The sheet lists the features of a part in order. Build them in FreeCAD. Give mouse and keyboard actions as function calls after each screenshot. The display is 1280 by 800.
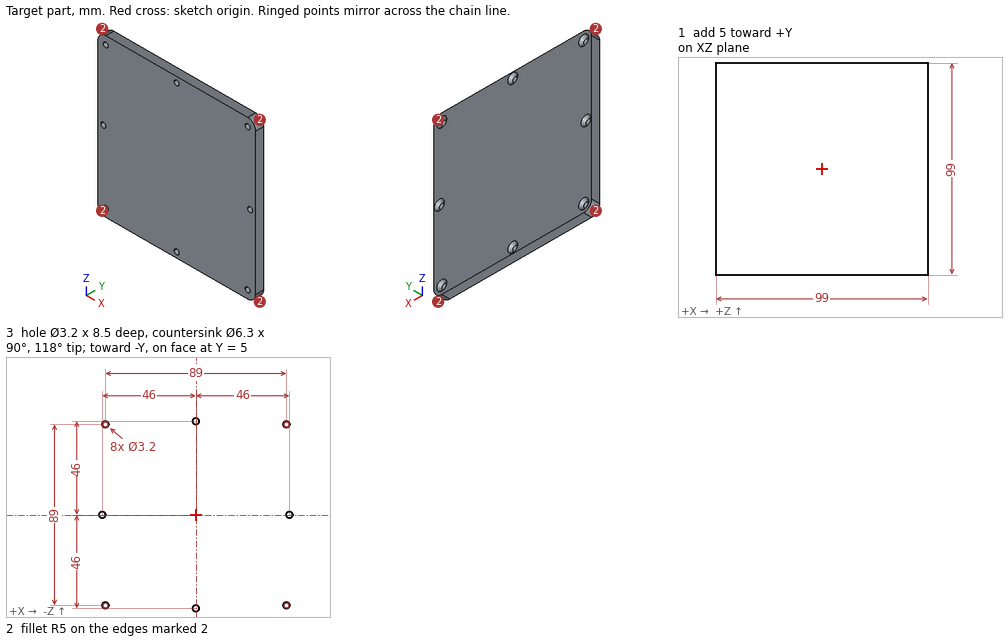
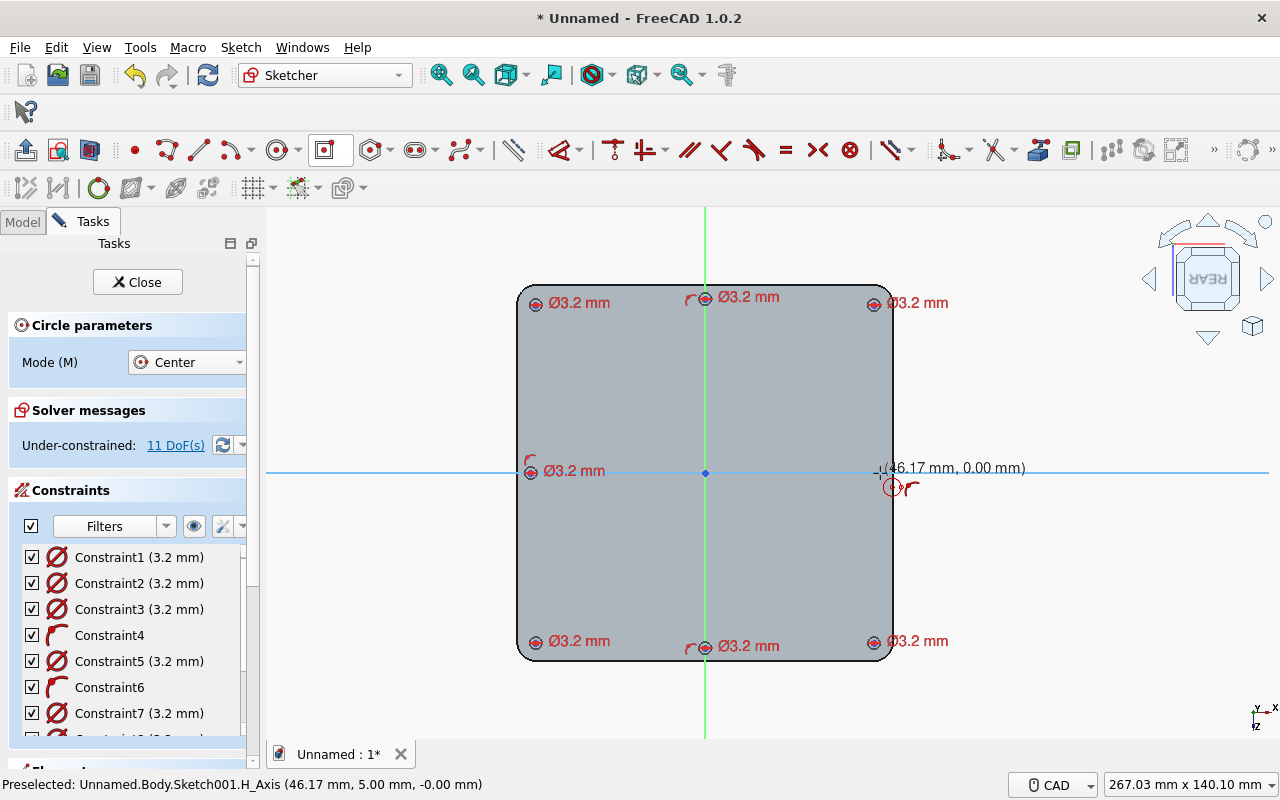
click(880, 473)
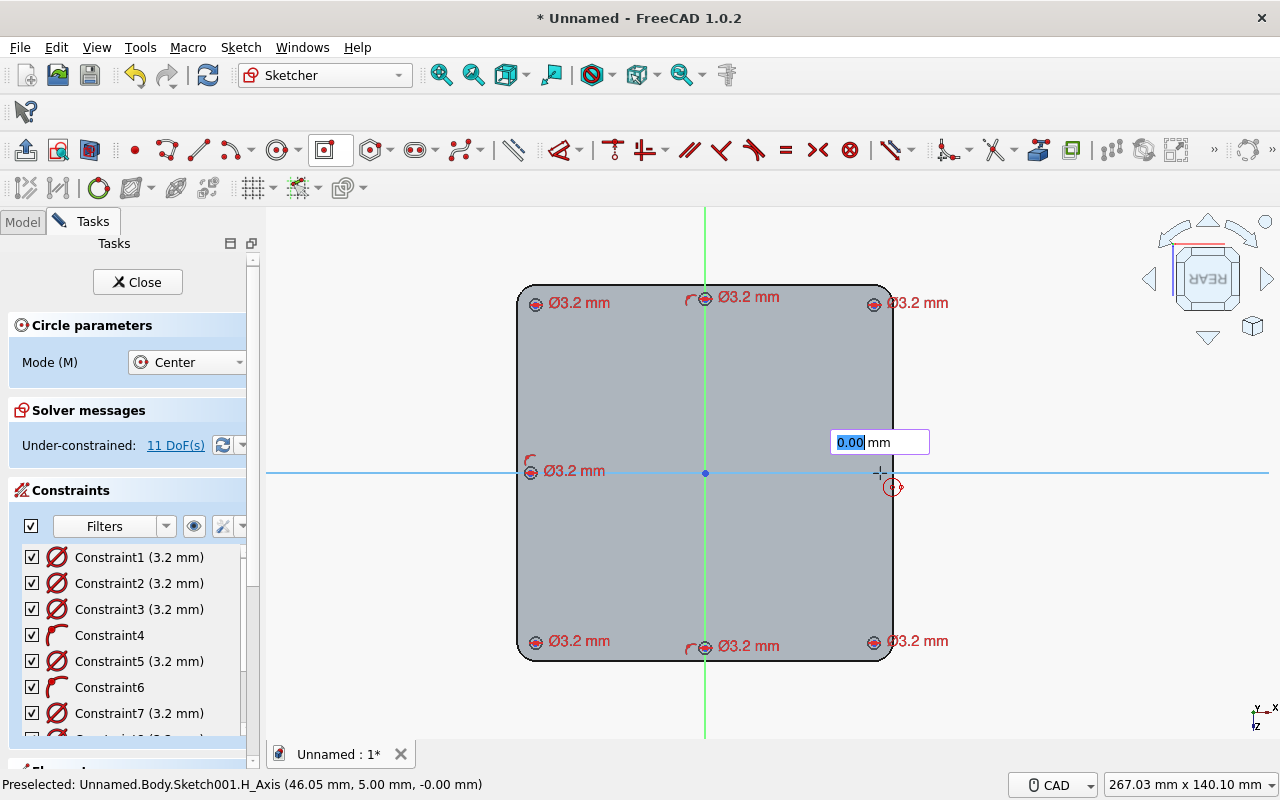
scroll(878, 479, up, 6)
move(876, 477)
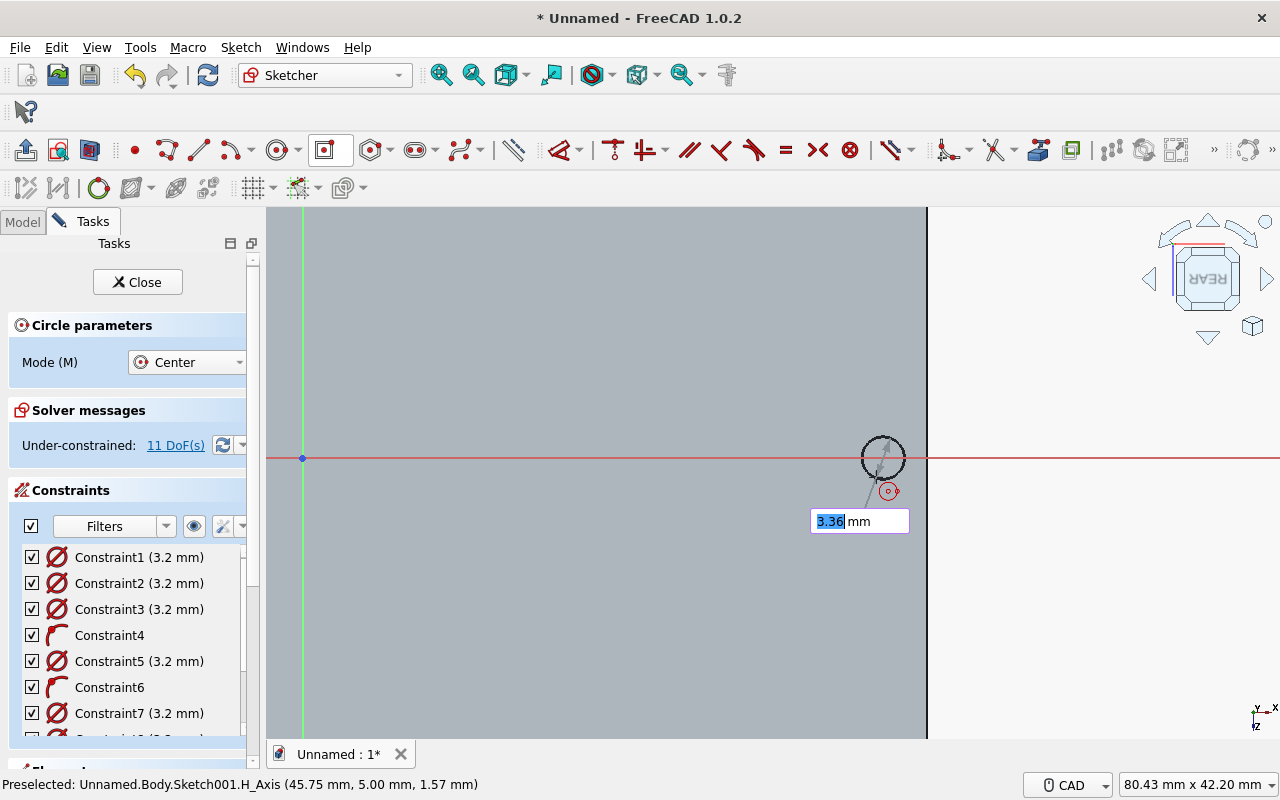
text(3.2)
key(Return)
key(Escape)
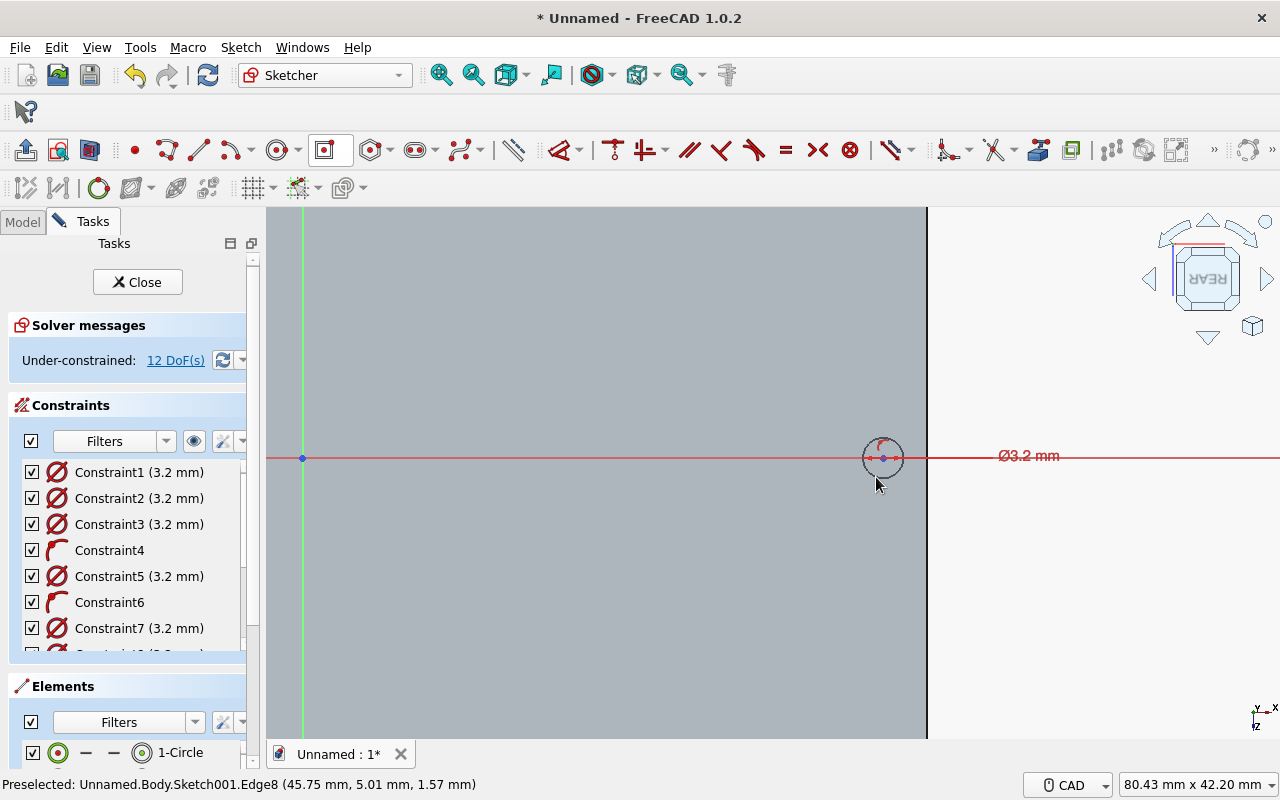
scroll(878, 479, down, 6)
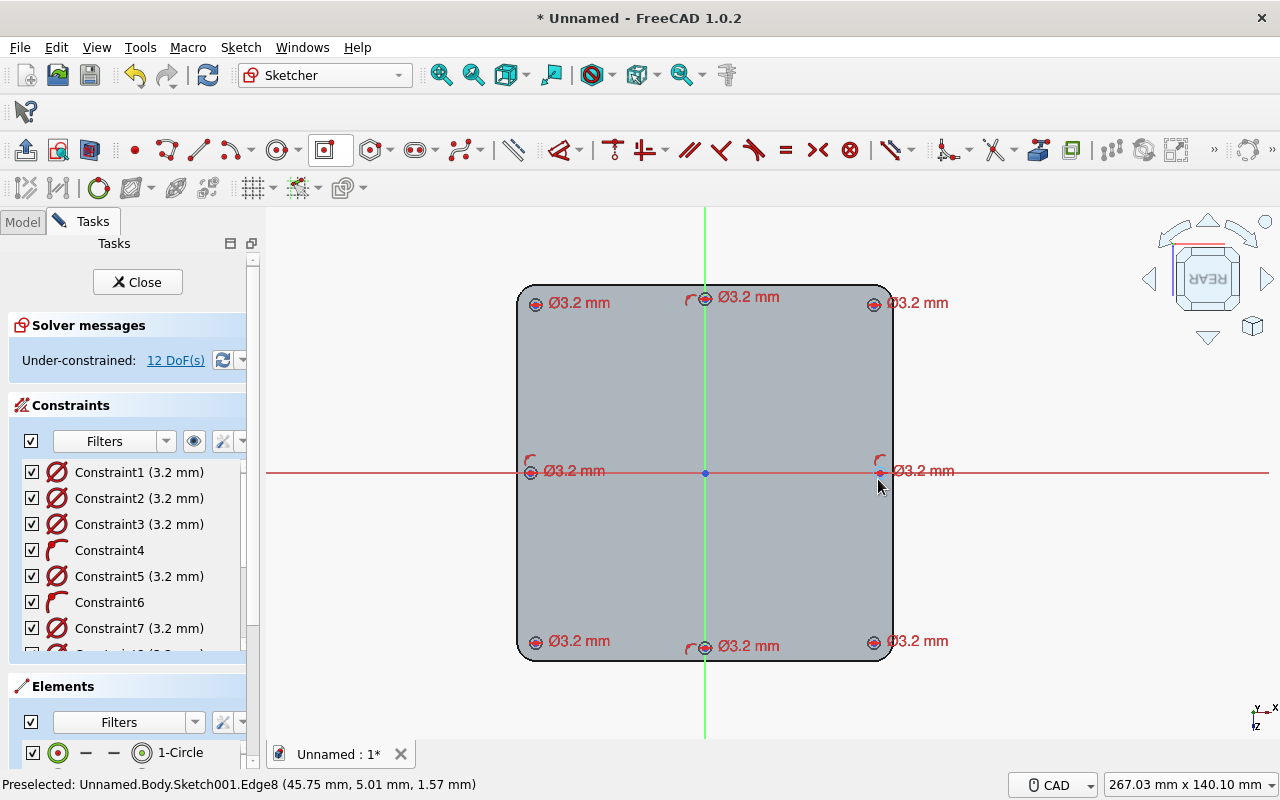
click(536, 305)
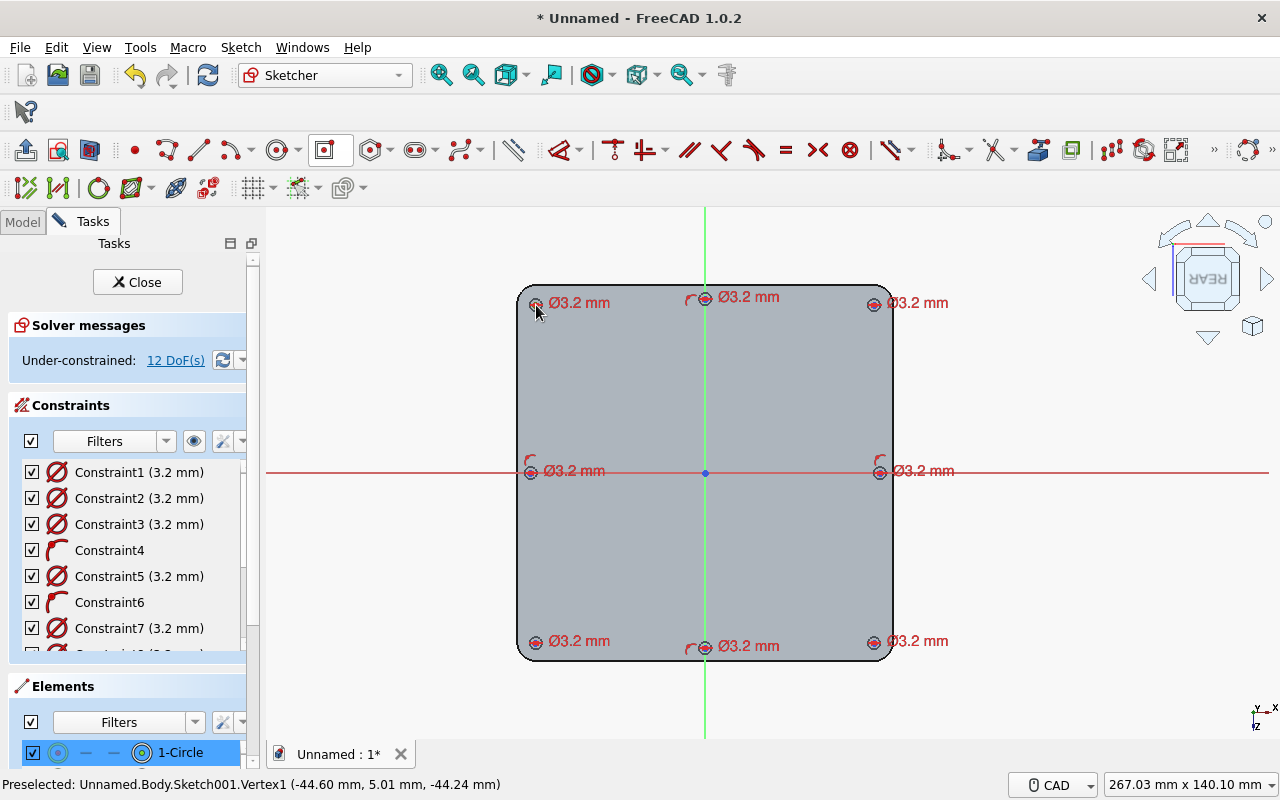
click(874, 305)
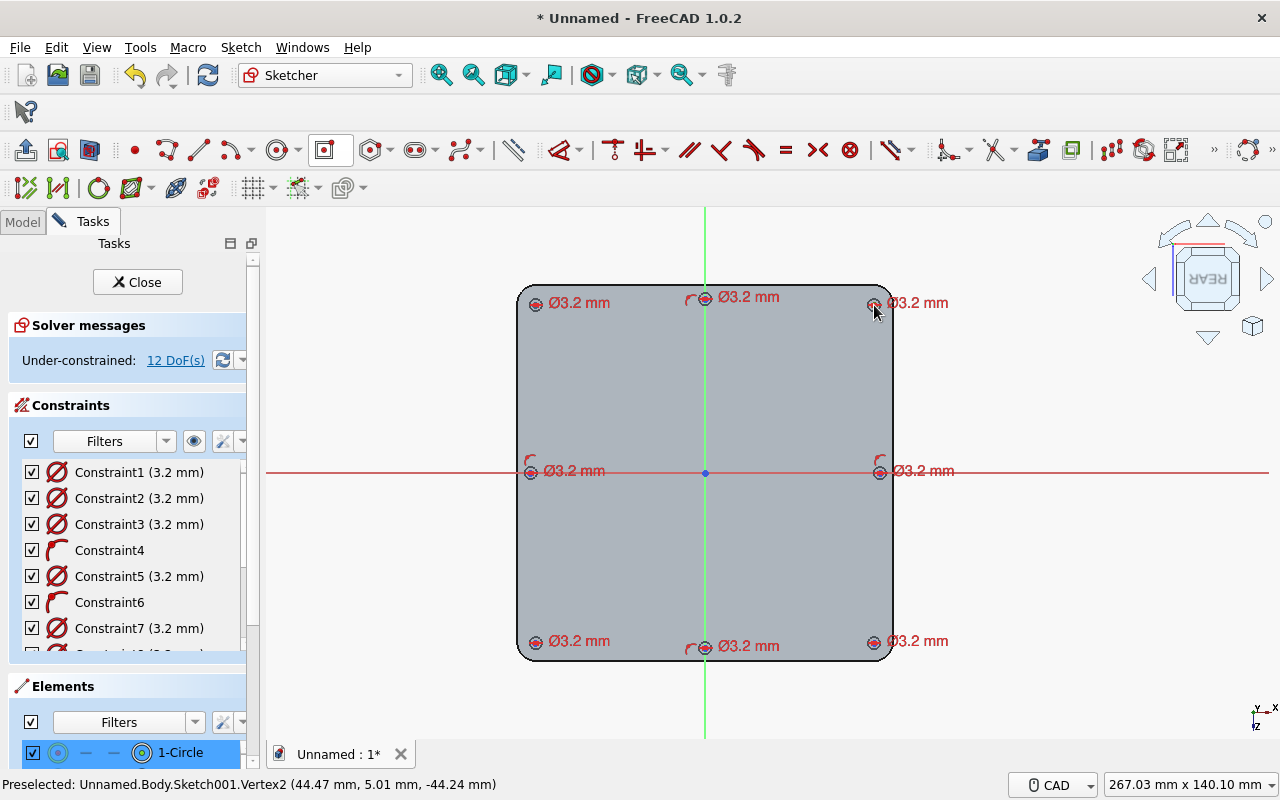
click(705, 609)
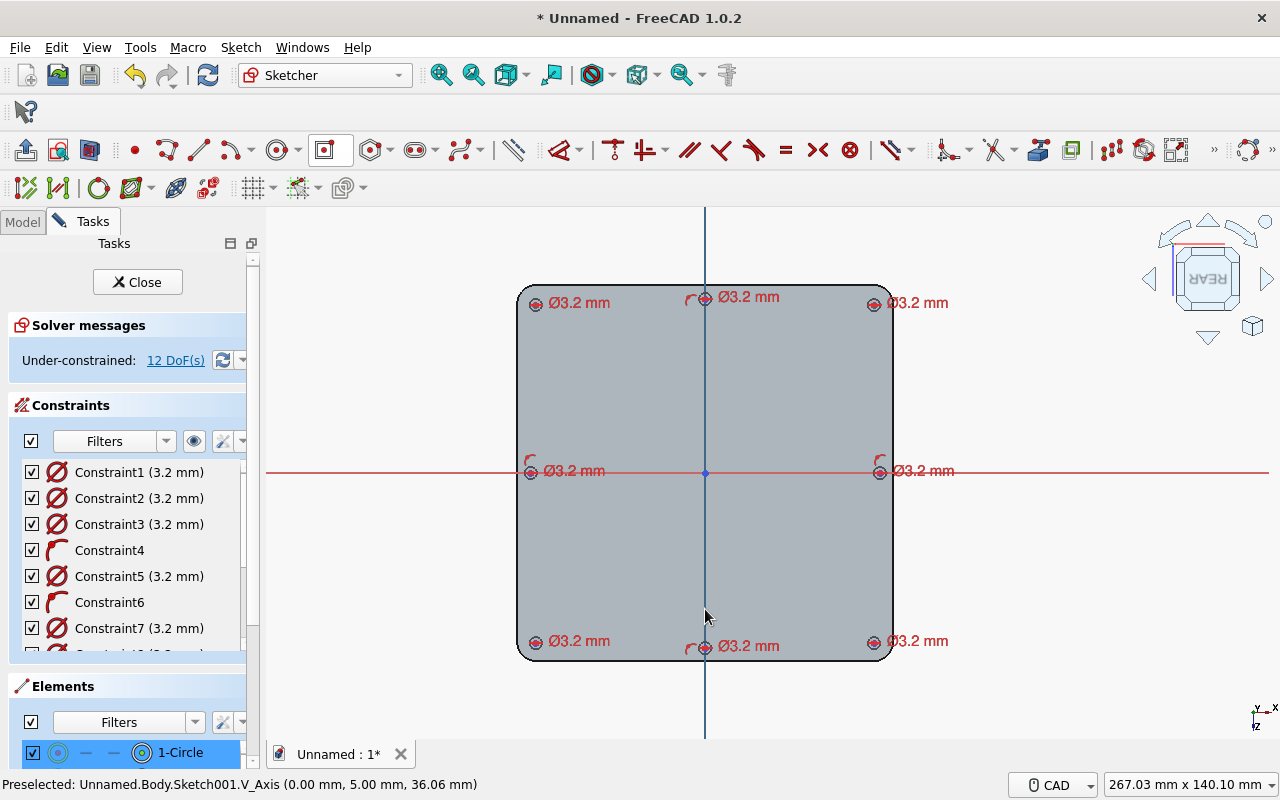
key(s)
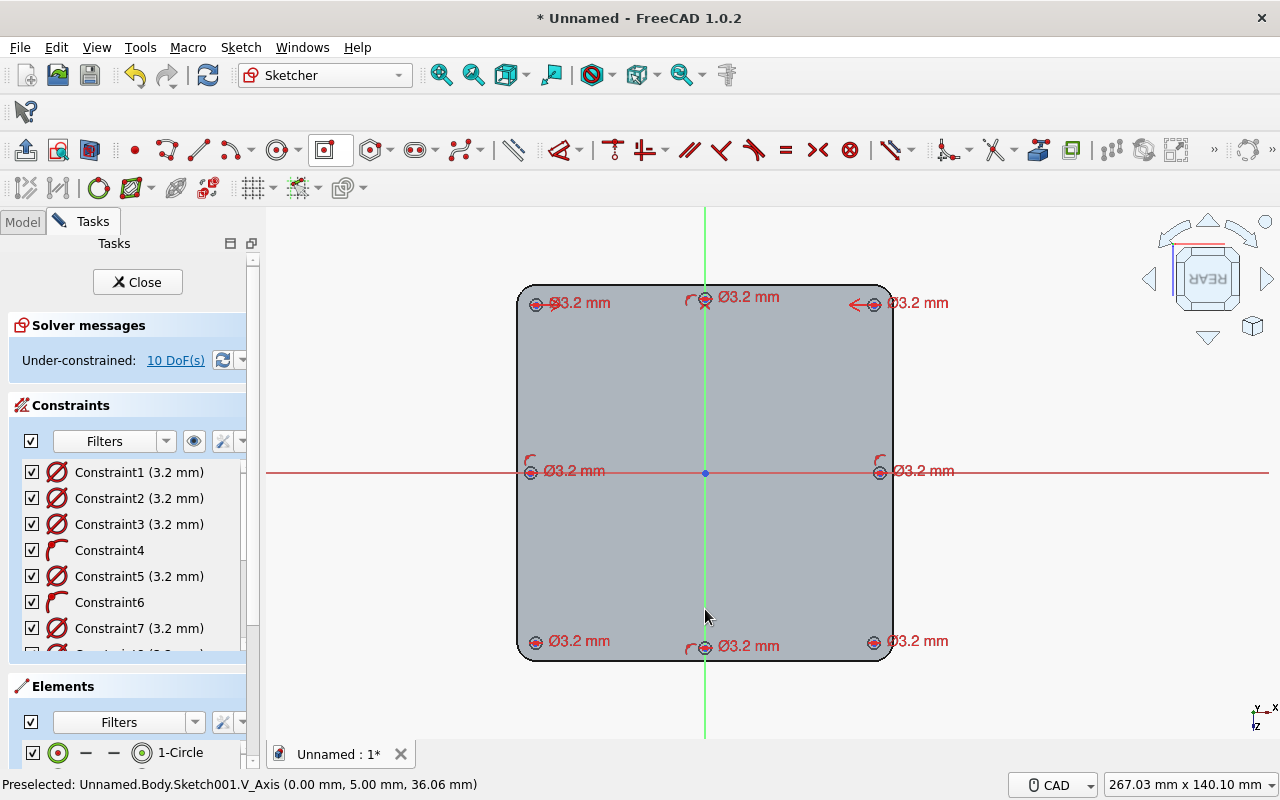
click(536, 305)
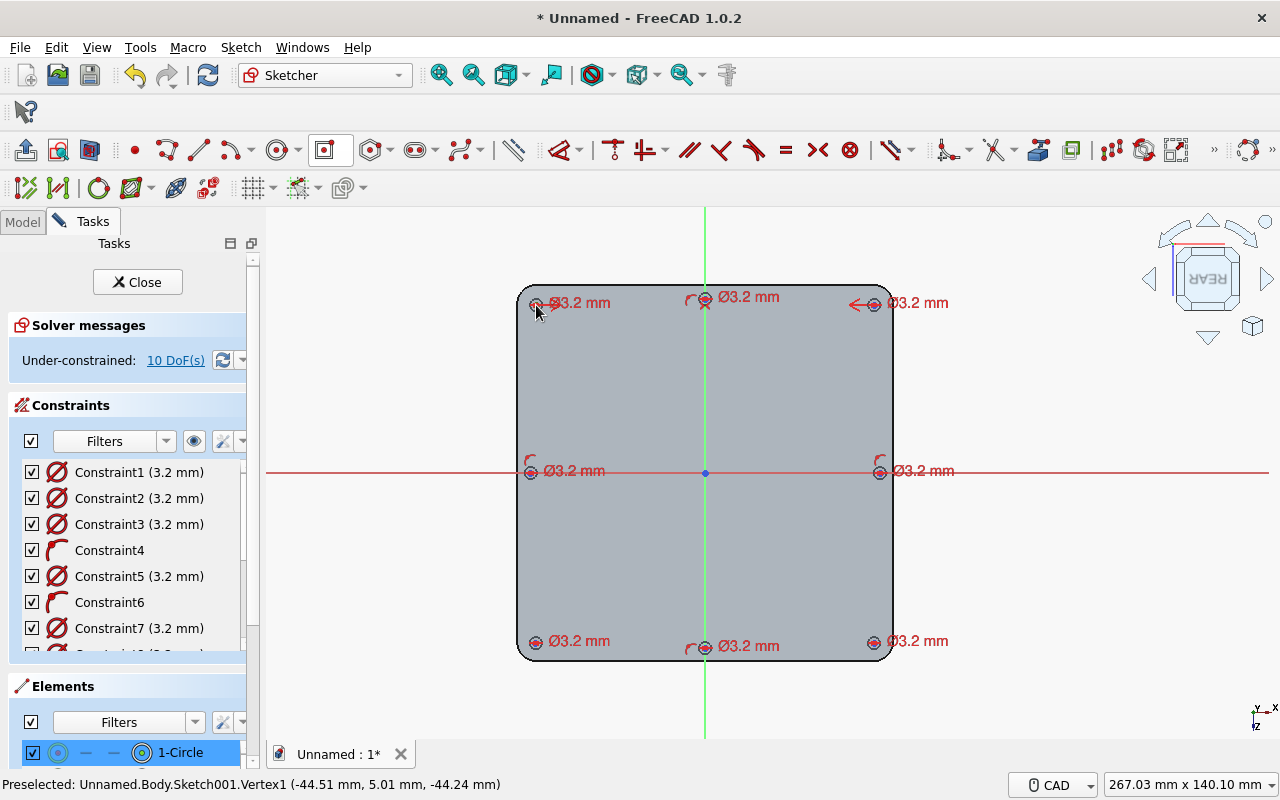
click(536, 643)